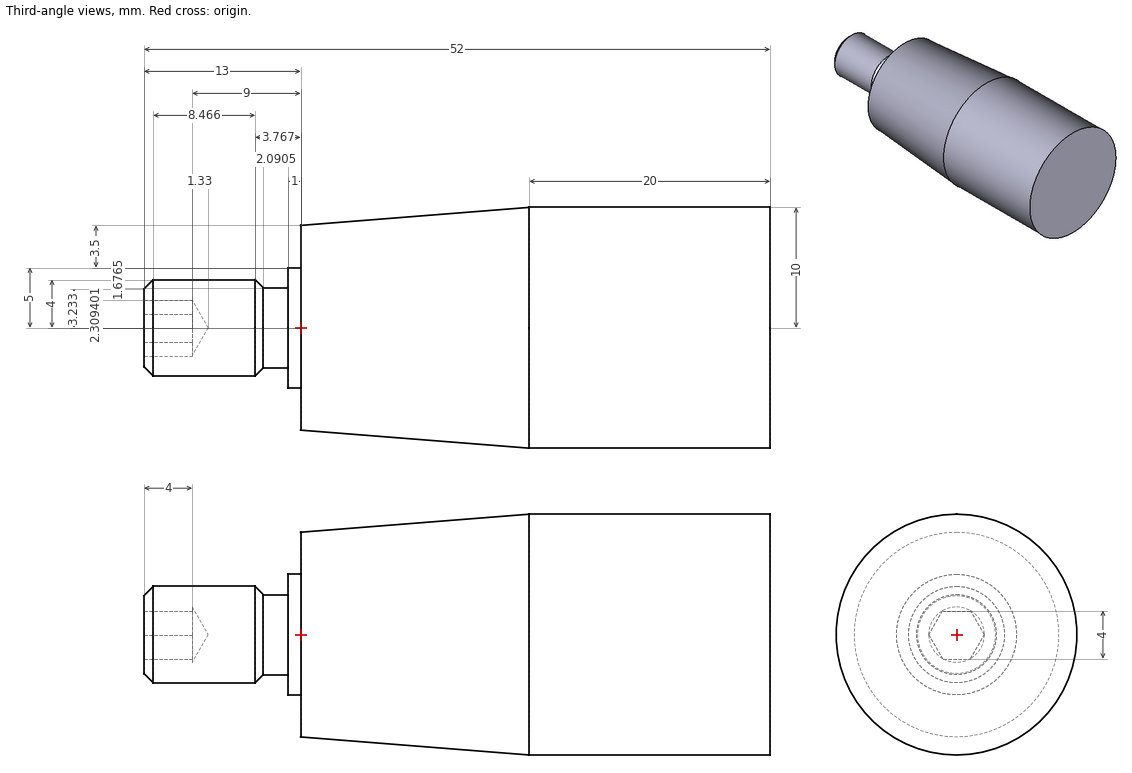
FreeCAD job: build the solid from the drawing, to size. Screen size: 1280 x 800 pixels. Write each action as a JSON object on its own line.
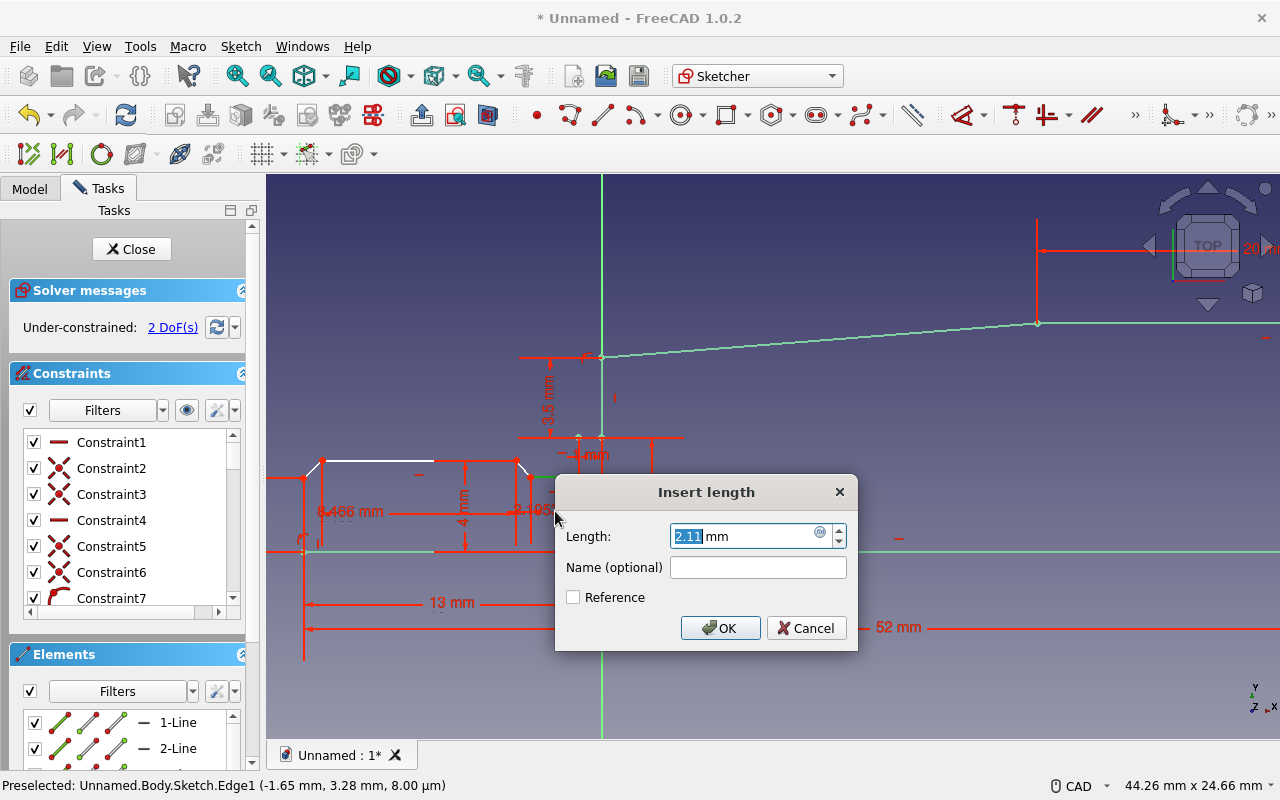
{"action": "type", "text": "2.0905"}
{"action": "key", "text": "Return"}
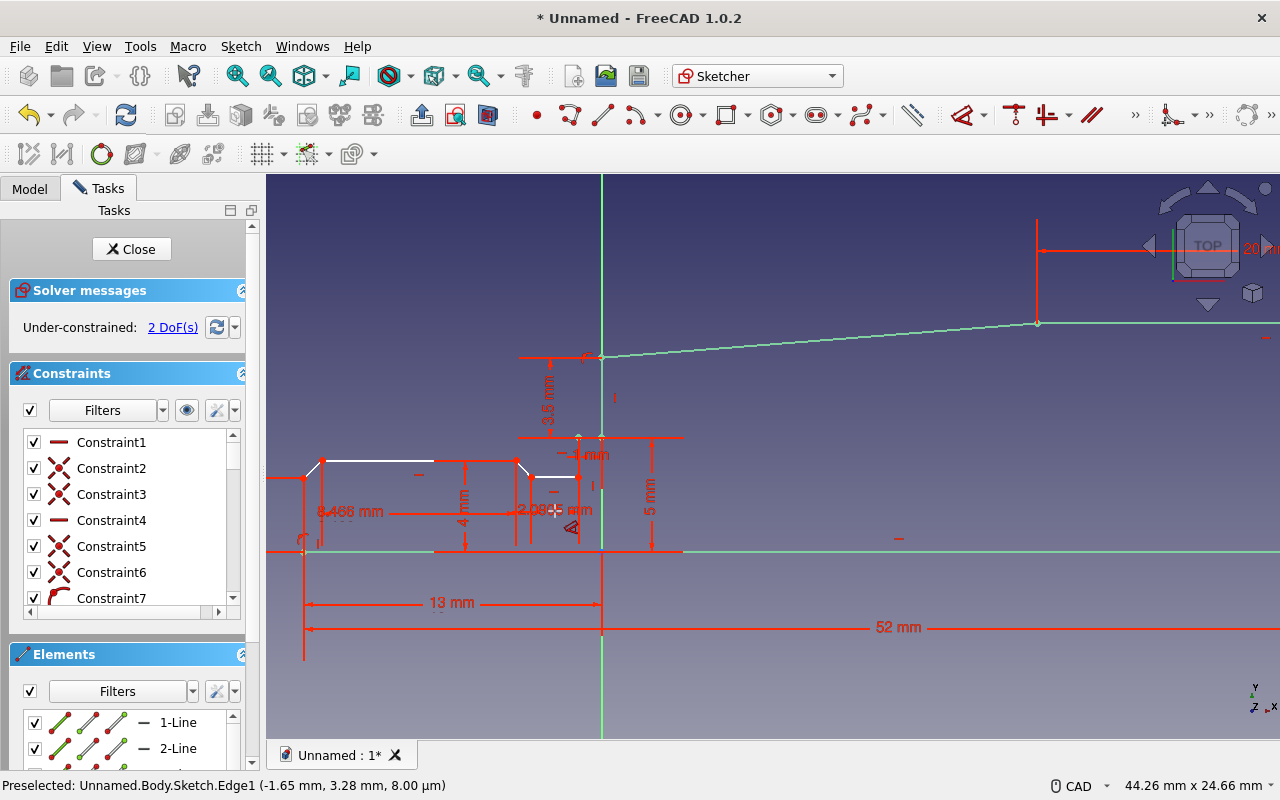
{"action": "left_click", "coordinate": [579, 450]}
{"action": "left_click", "coordinate": [497, 444]}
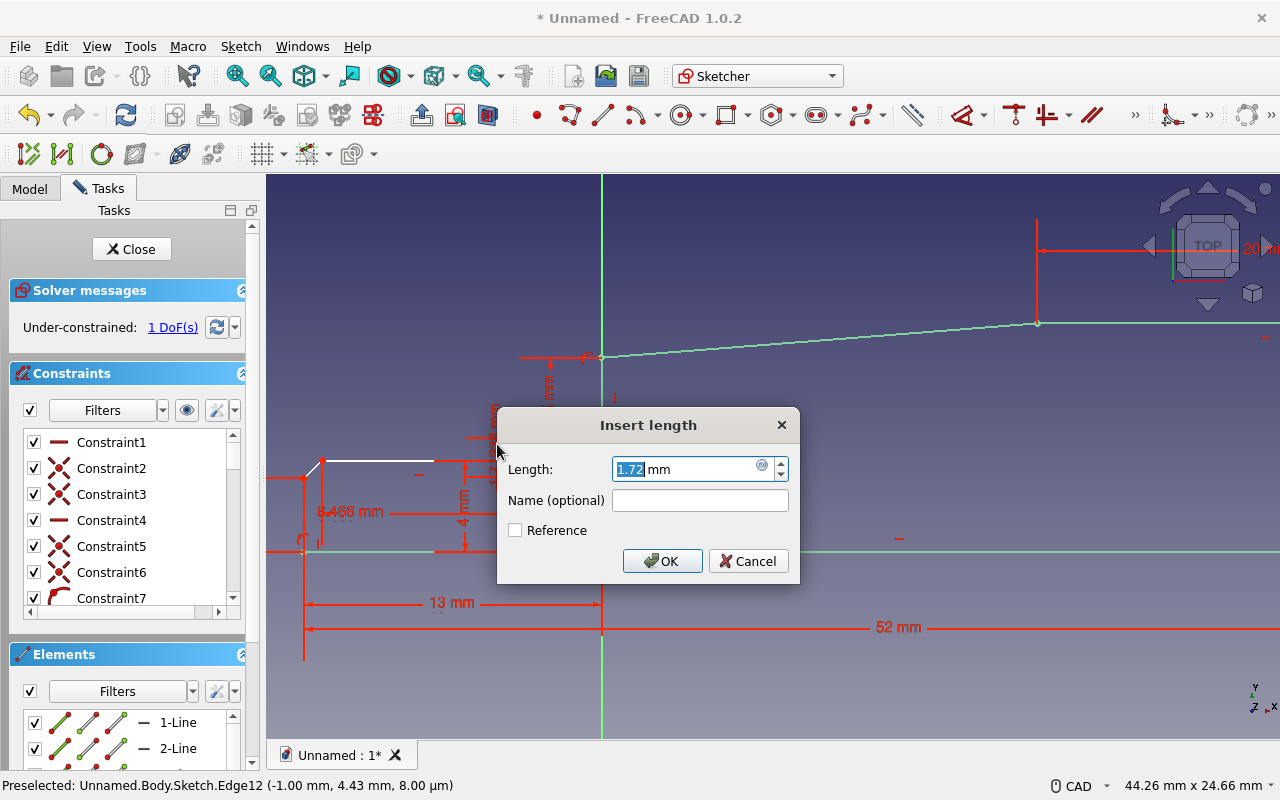
{"action": "type", "text": "1.6765"}
{"action": "key", "text": "Return"}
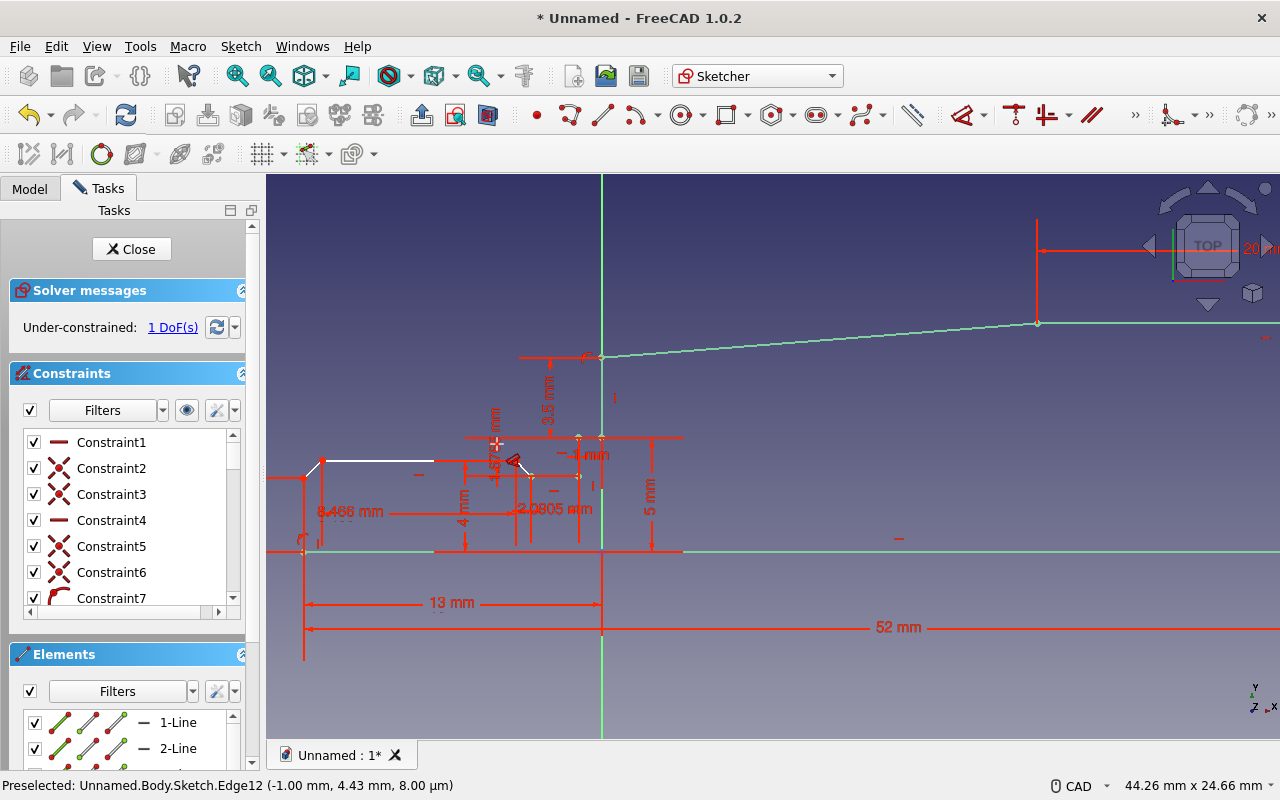
{"action": "left_click", "coordinate": [516, 461]}
{"action": "left_click", "coordinate": [559, 586]}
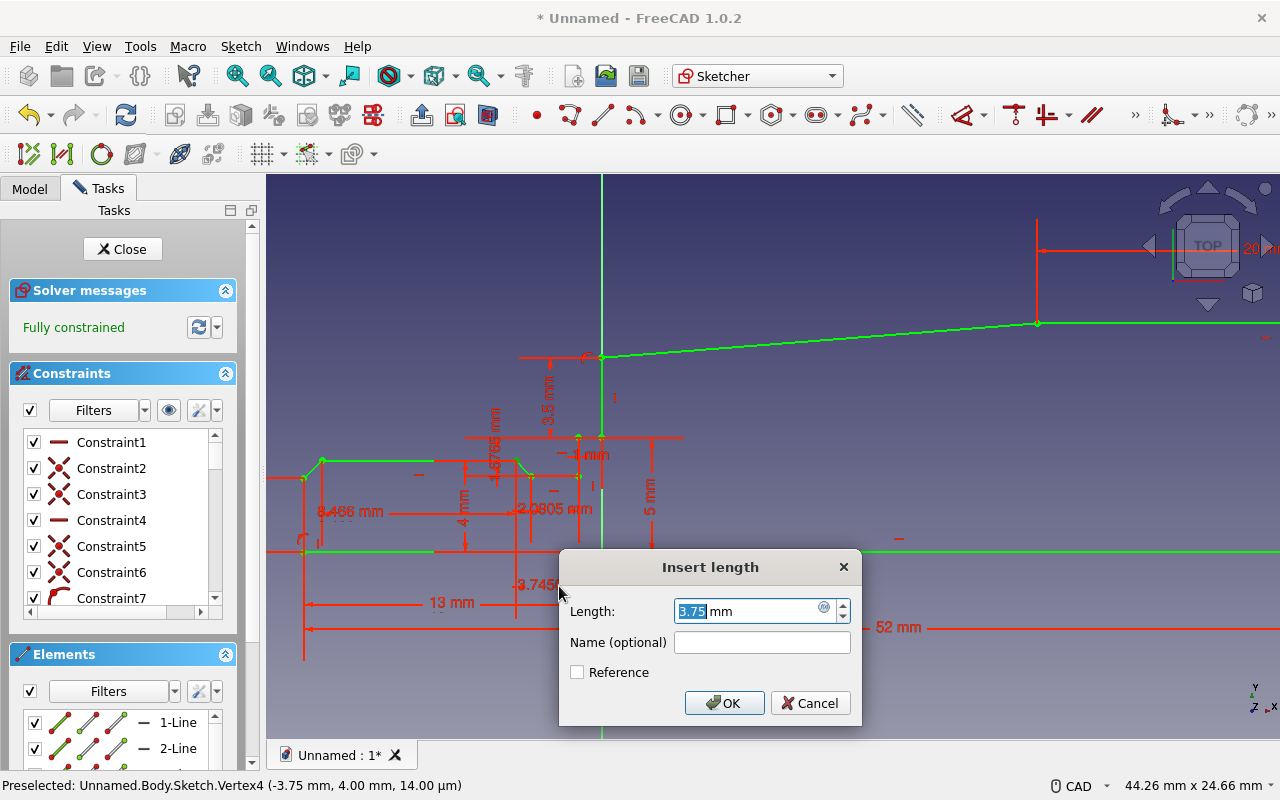
{"action": "type", "text": "3.767"}
{"action": "key", "text": "Return"}
{"action": "key", "text": "Escape"}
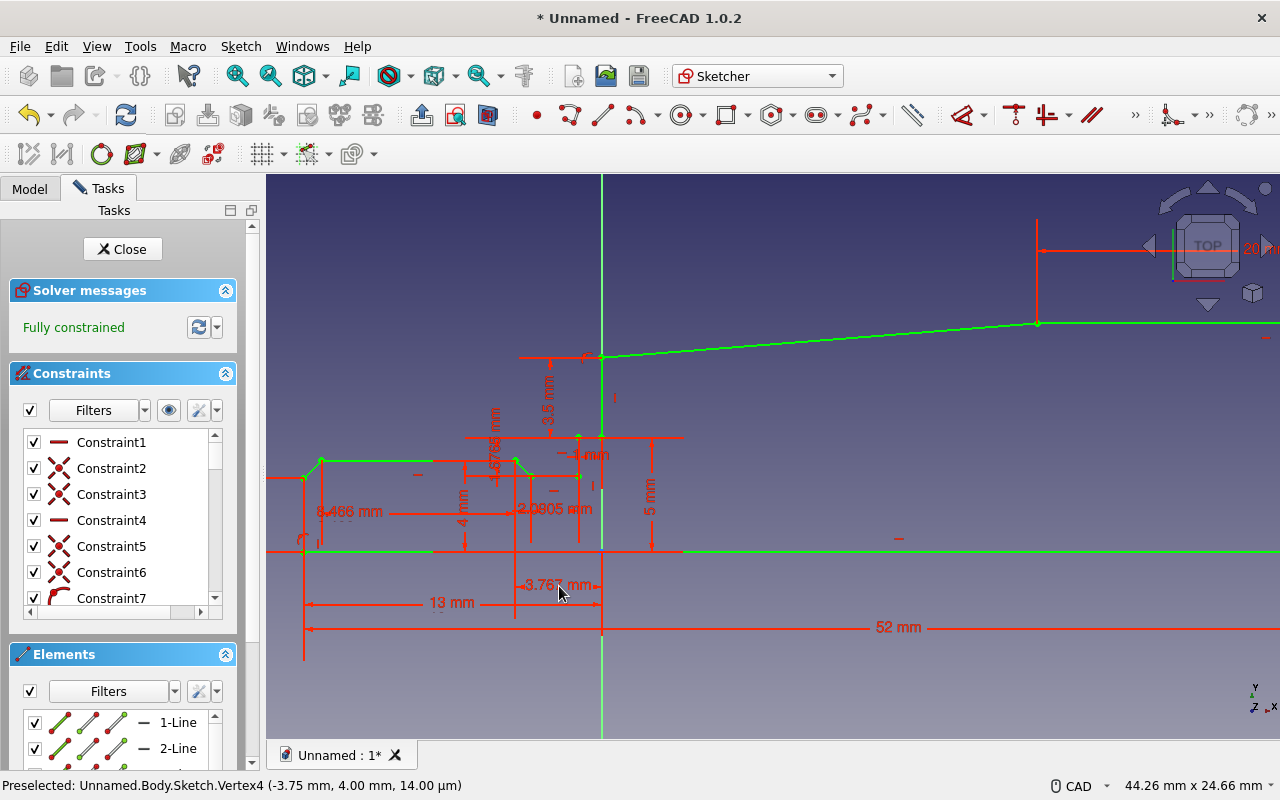
{"action": "left_click", "coordinate": [123, 249]}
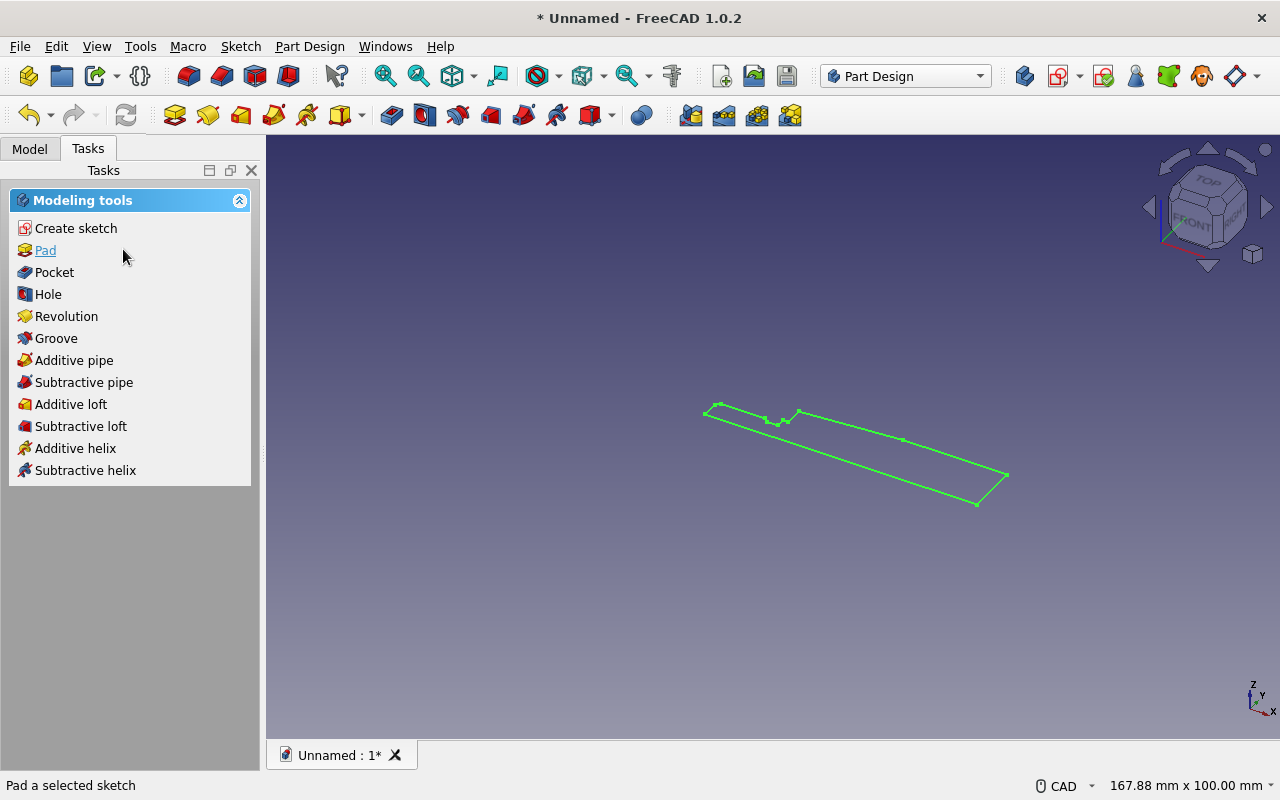
{"action": "left_click", "coordinate": [208, 116]}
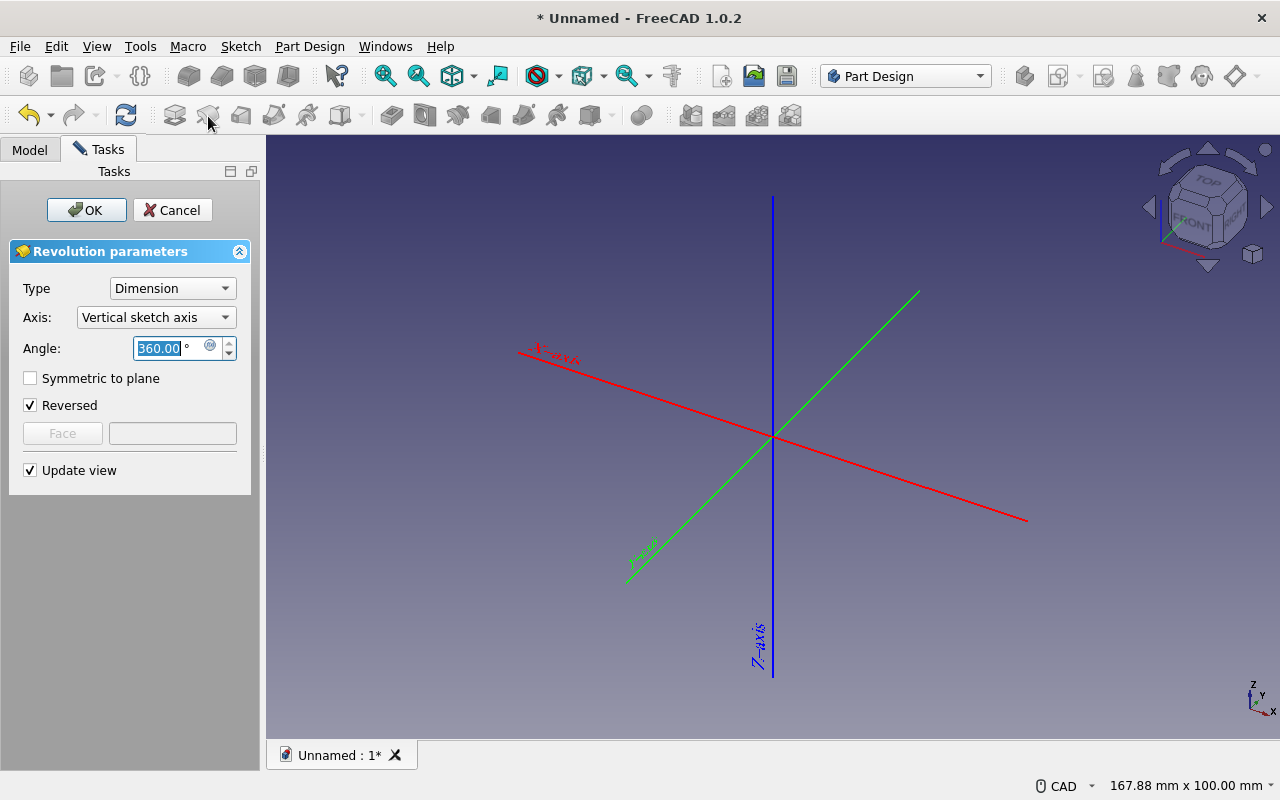
{"action": "left_click", "coordinate": [157, 318]}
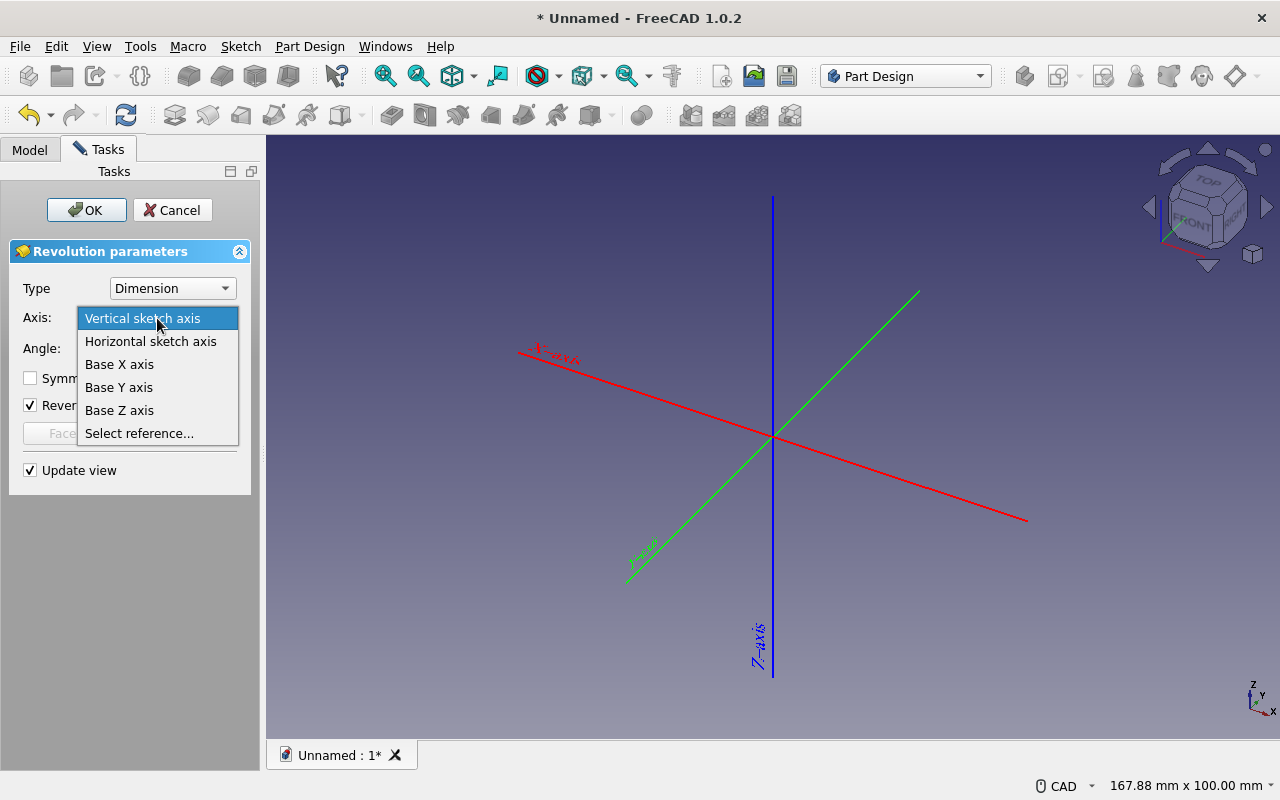
{"action": "left_click", "coordinate": [156, 342]}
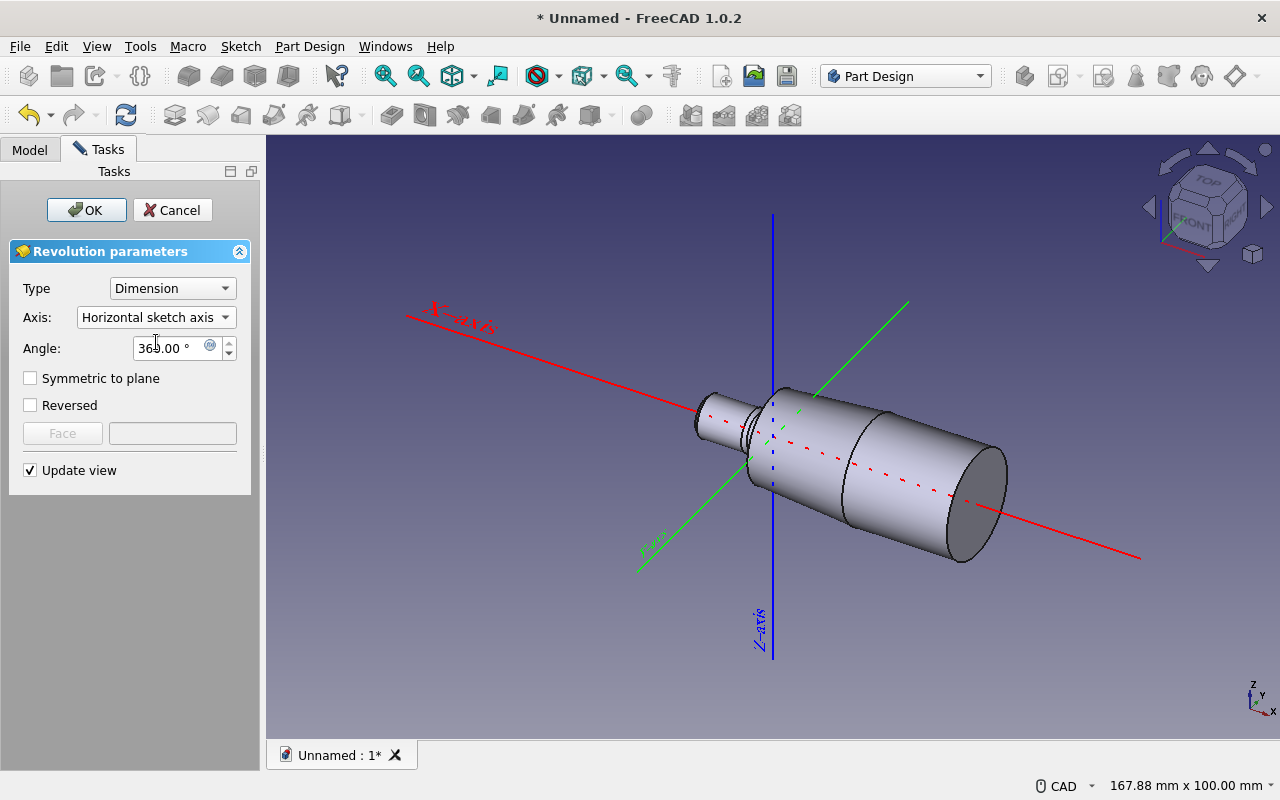
{"action": "left_click", "coordinate": [87, 210]}